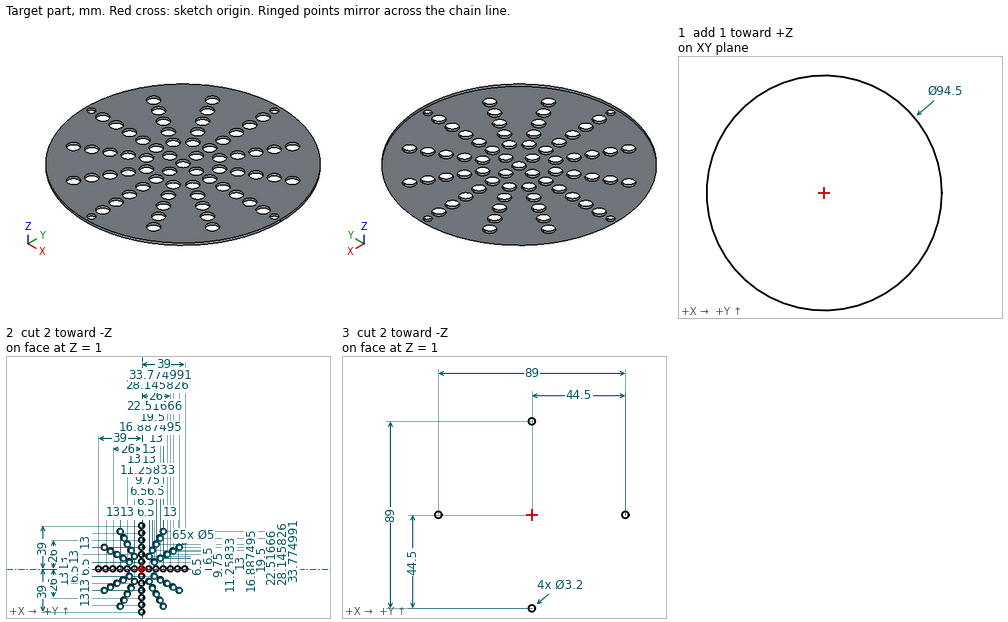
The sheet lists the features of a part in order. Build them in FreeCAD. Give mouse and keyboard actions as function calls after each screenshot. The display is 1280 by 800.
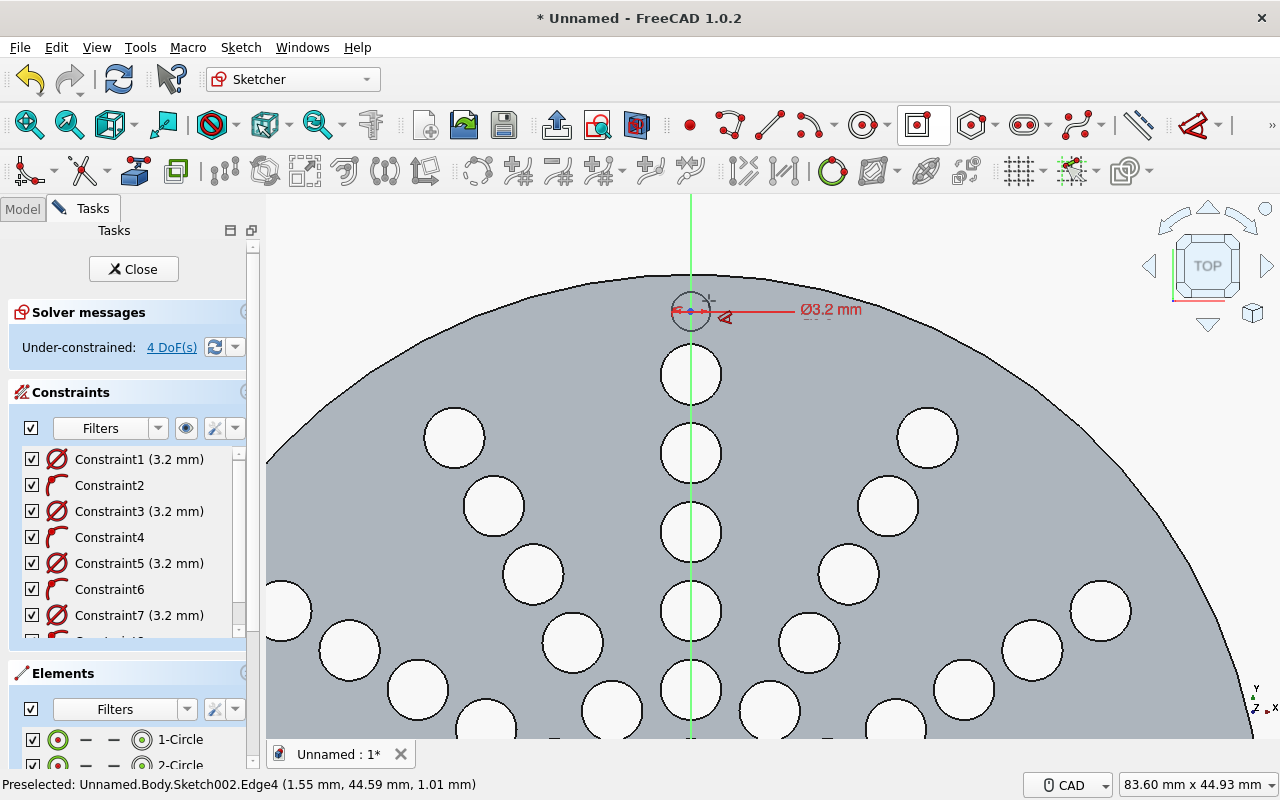
scroll(710, 302, down, 6)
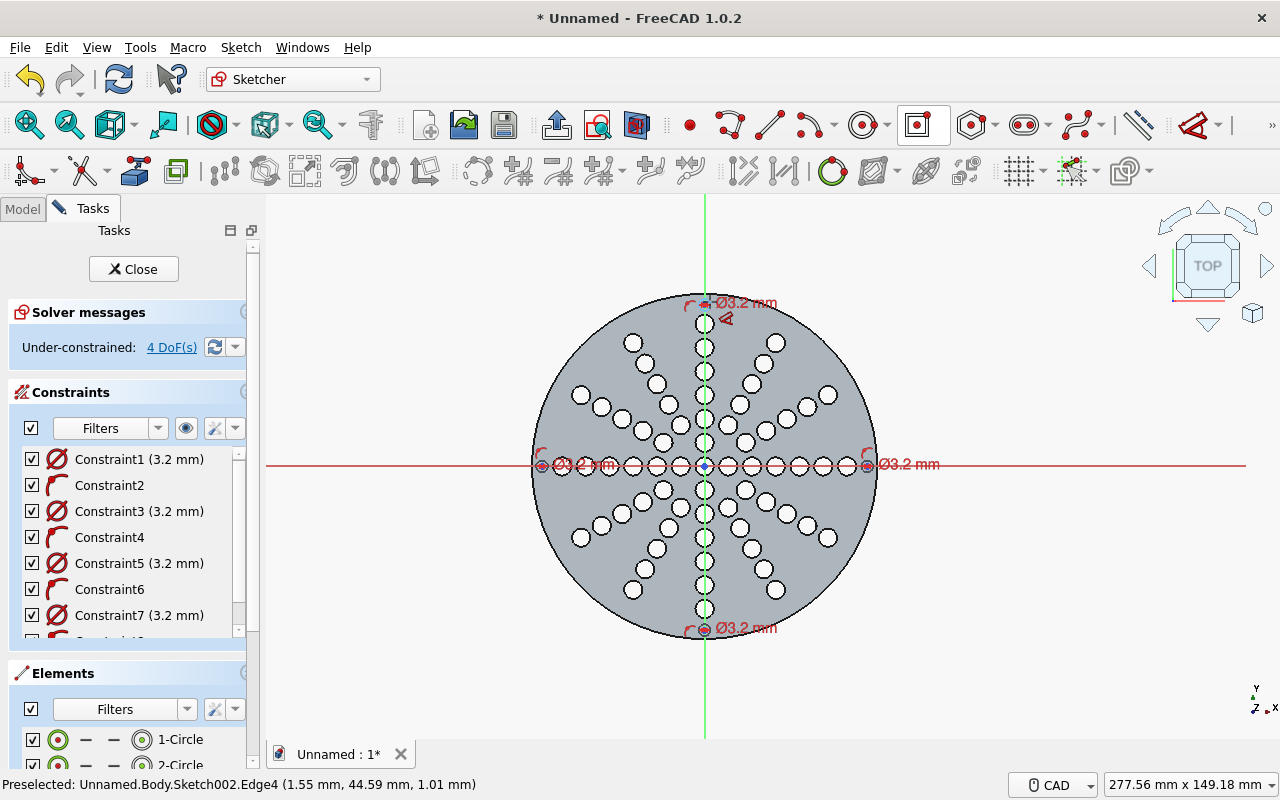
click(867, 466)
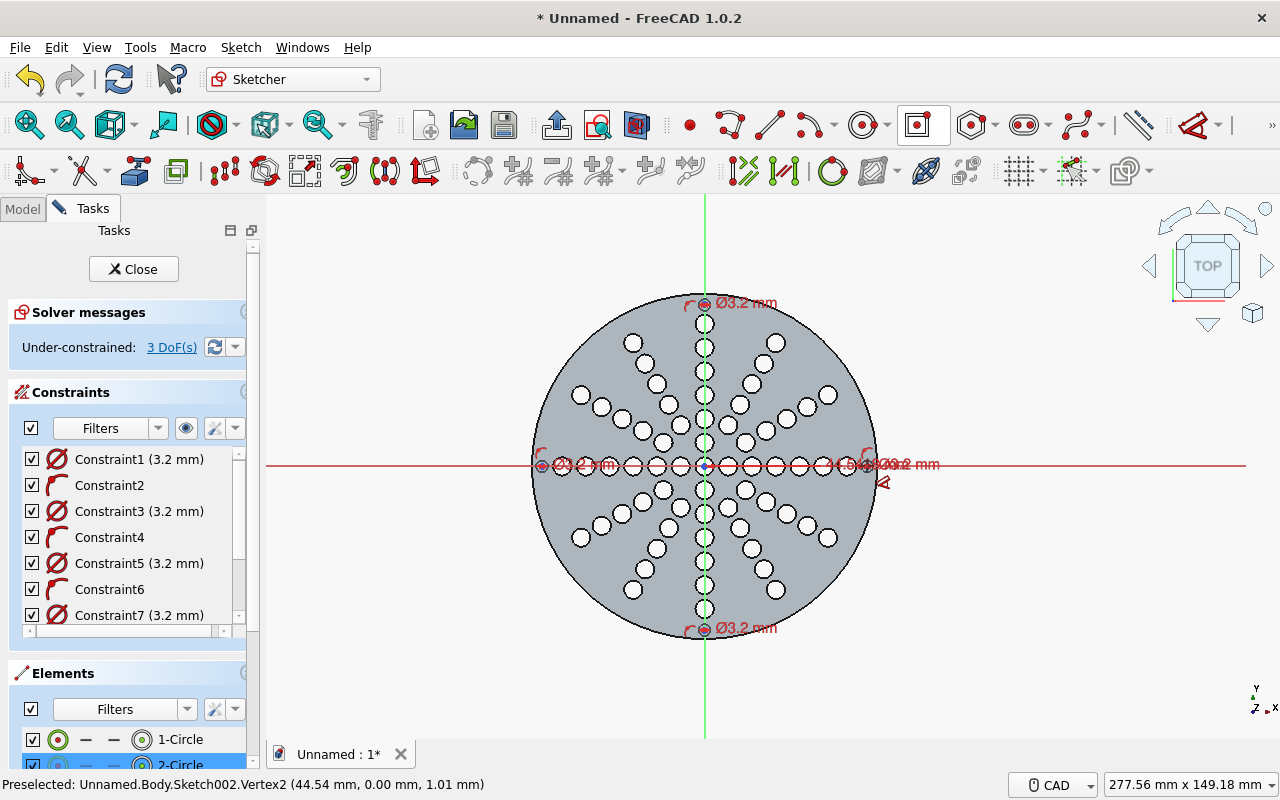
click(542, 466)
click(630, 500)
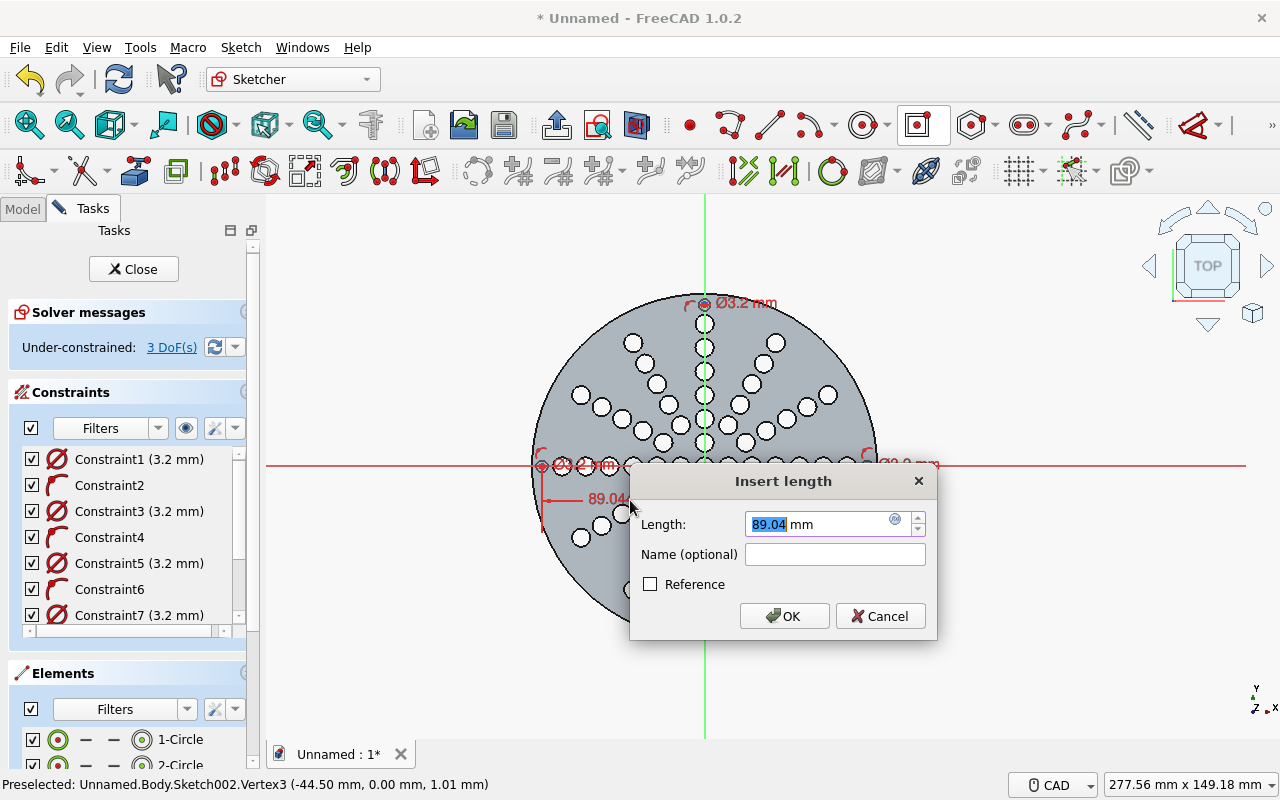
text(89)
key(Return)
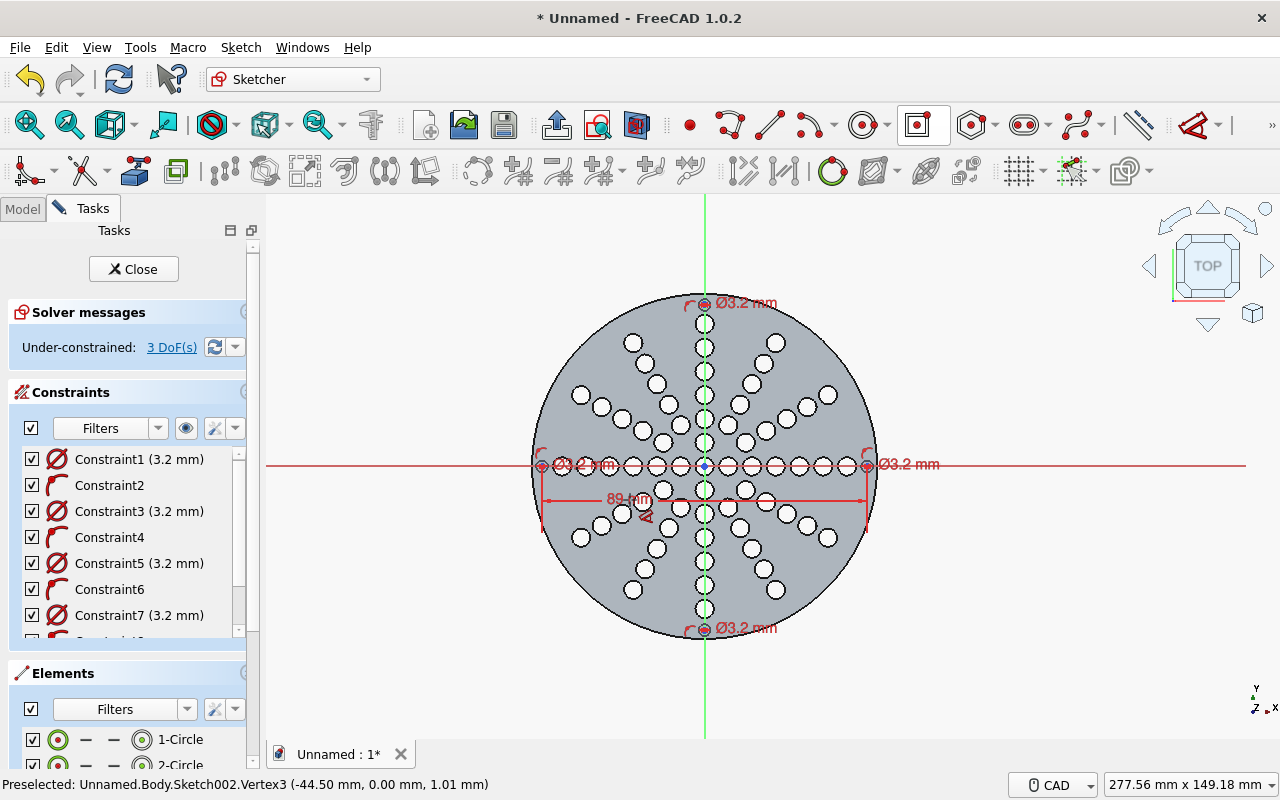
click(705, 630)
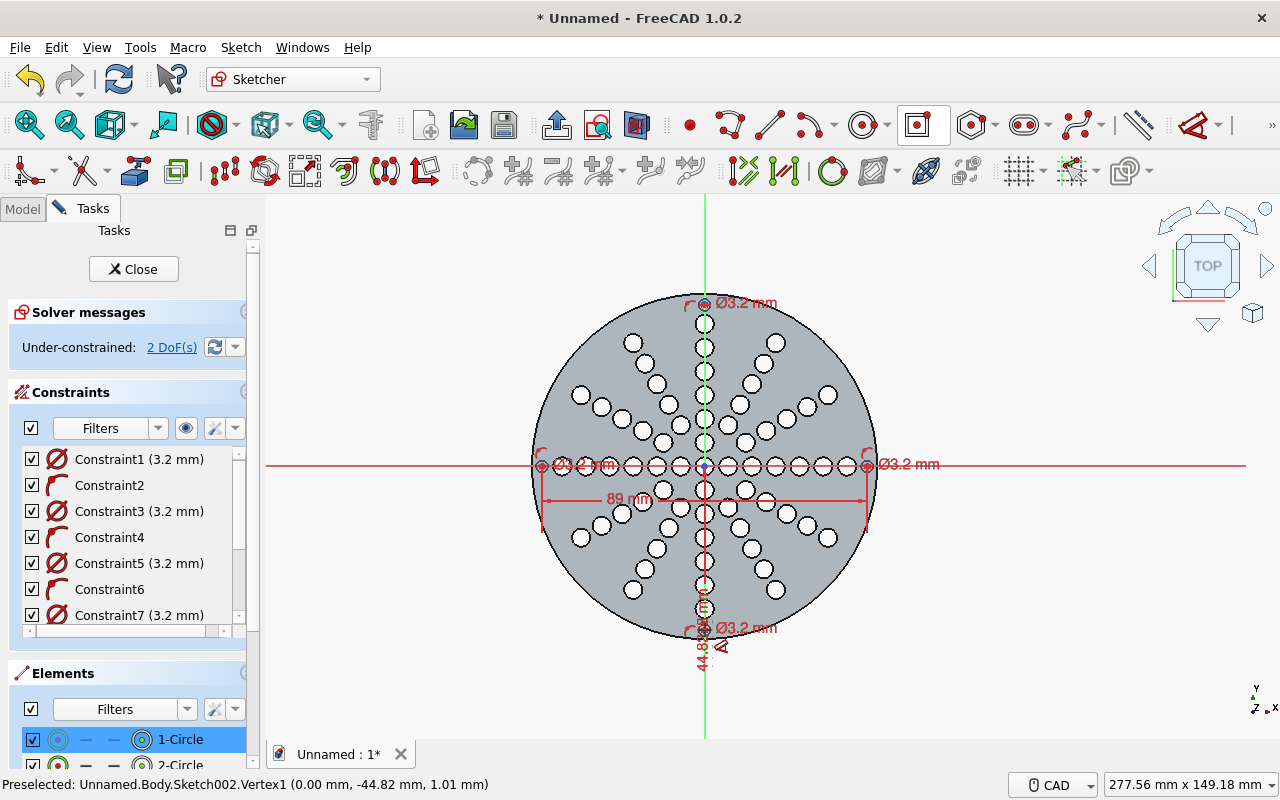
click(705, 305)
click(739, 393)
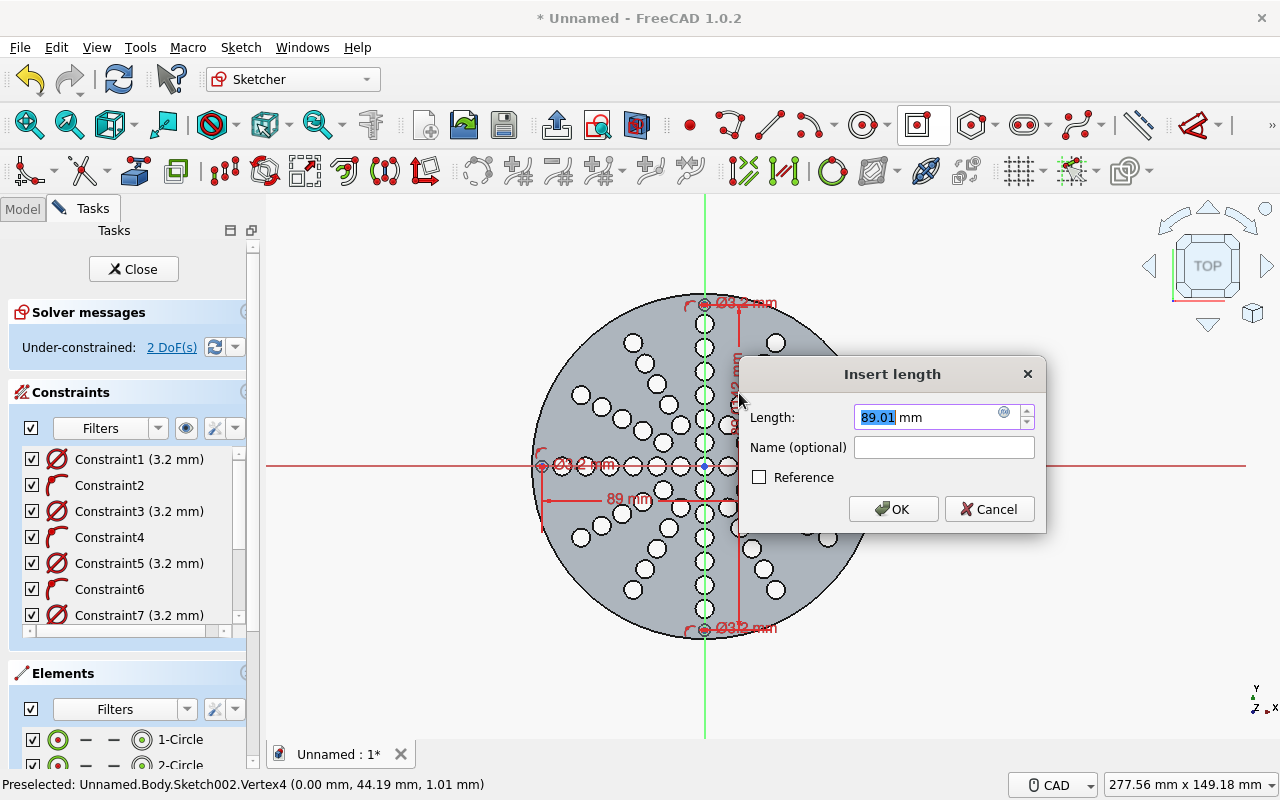
text(89)
key(Return)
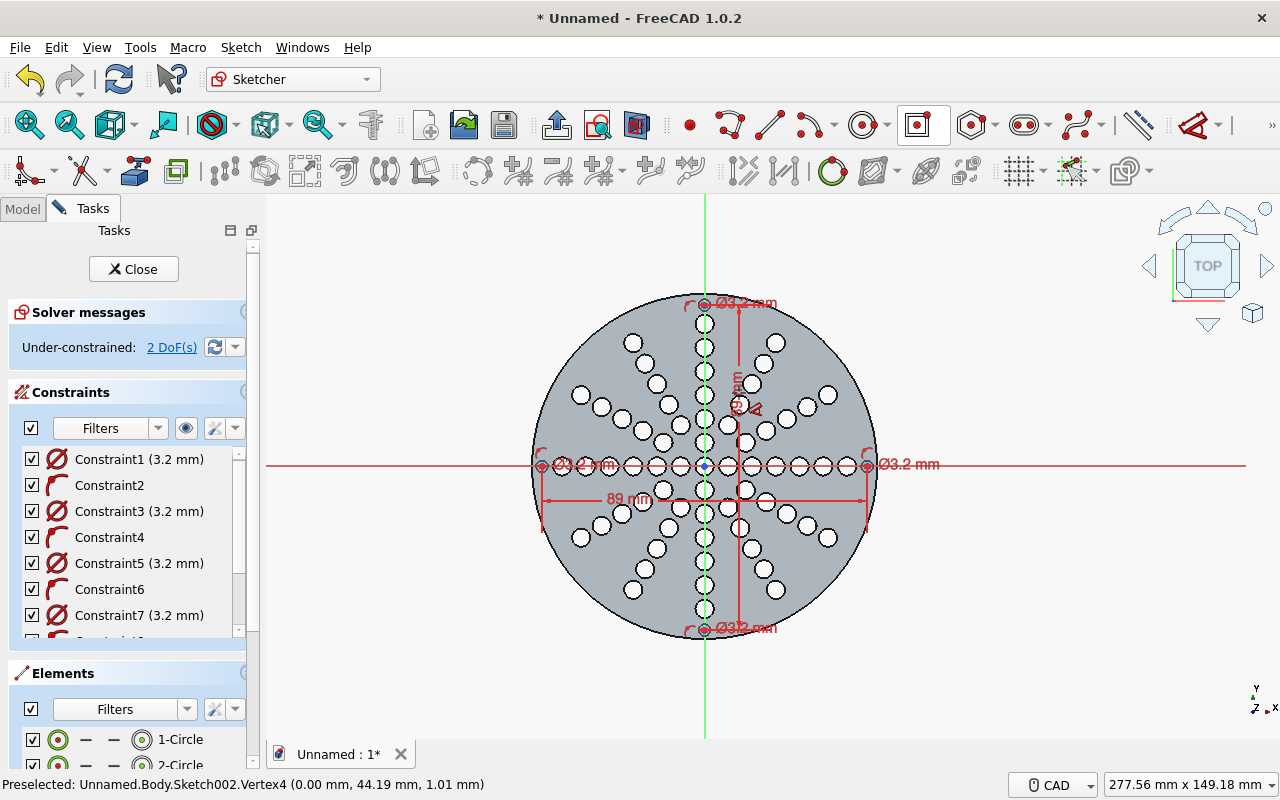
click(705, 630)
click(739, 548)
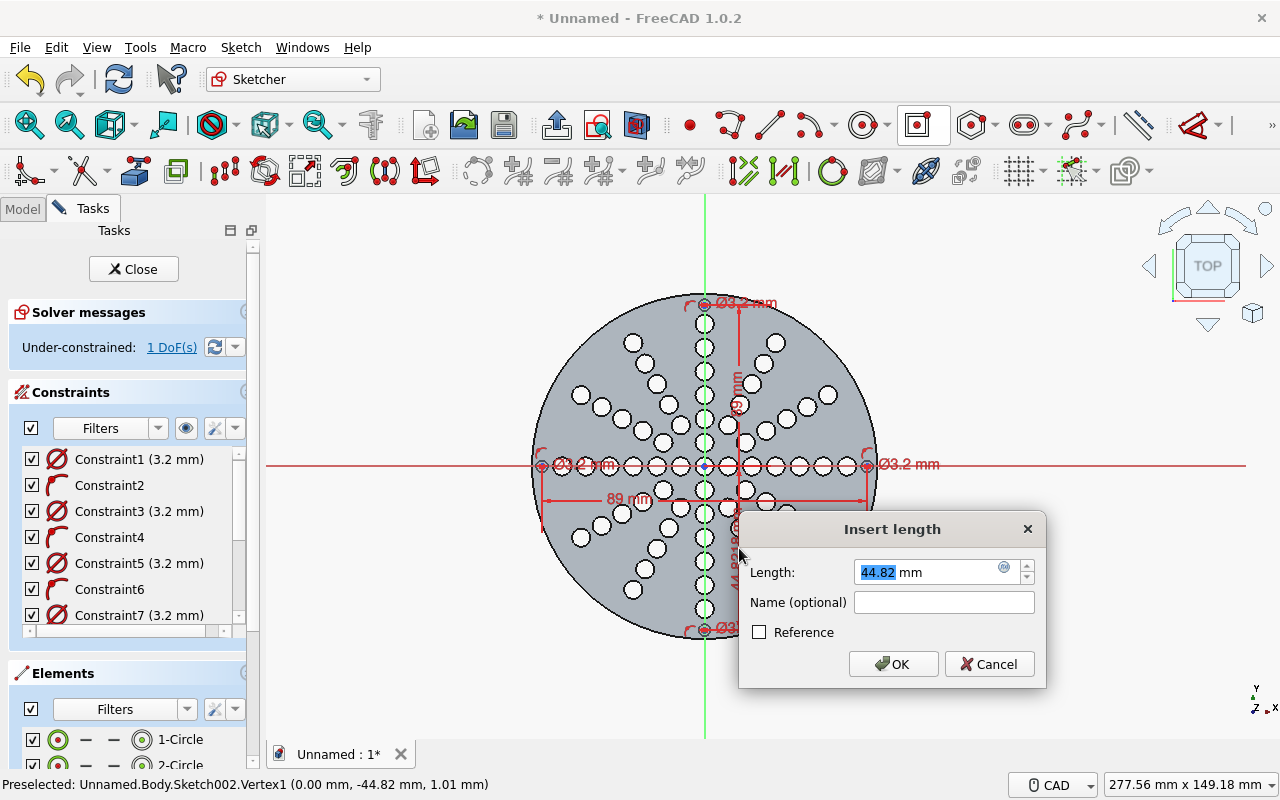
text(44.5)
key(Return)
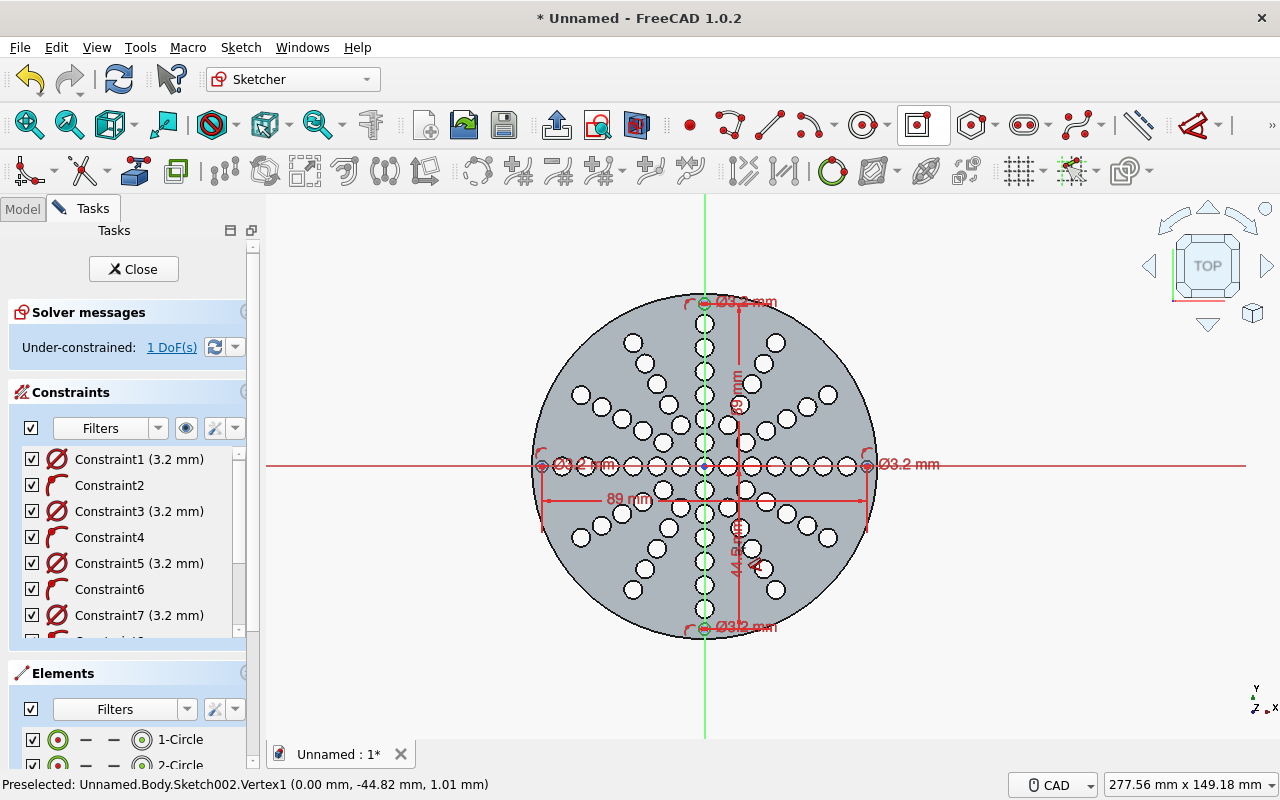
click(867, 466)
click(786, 500)